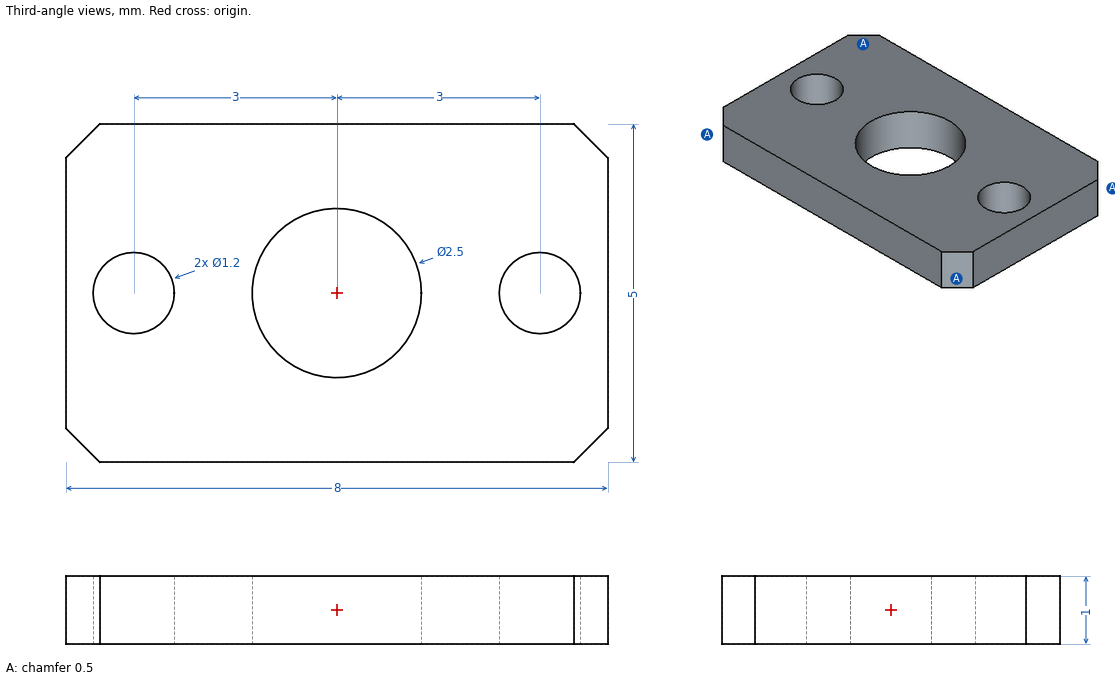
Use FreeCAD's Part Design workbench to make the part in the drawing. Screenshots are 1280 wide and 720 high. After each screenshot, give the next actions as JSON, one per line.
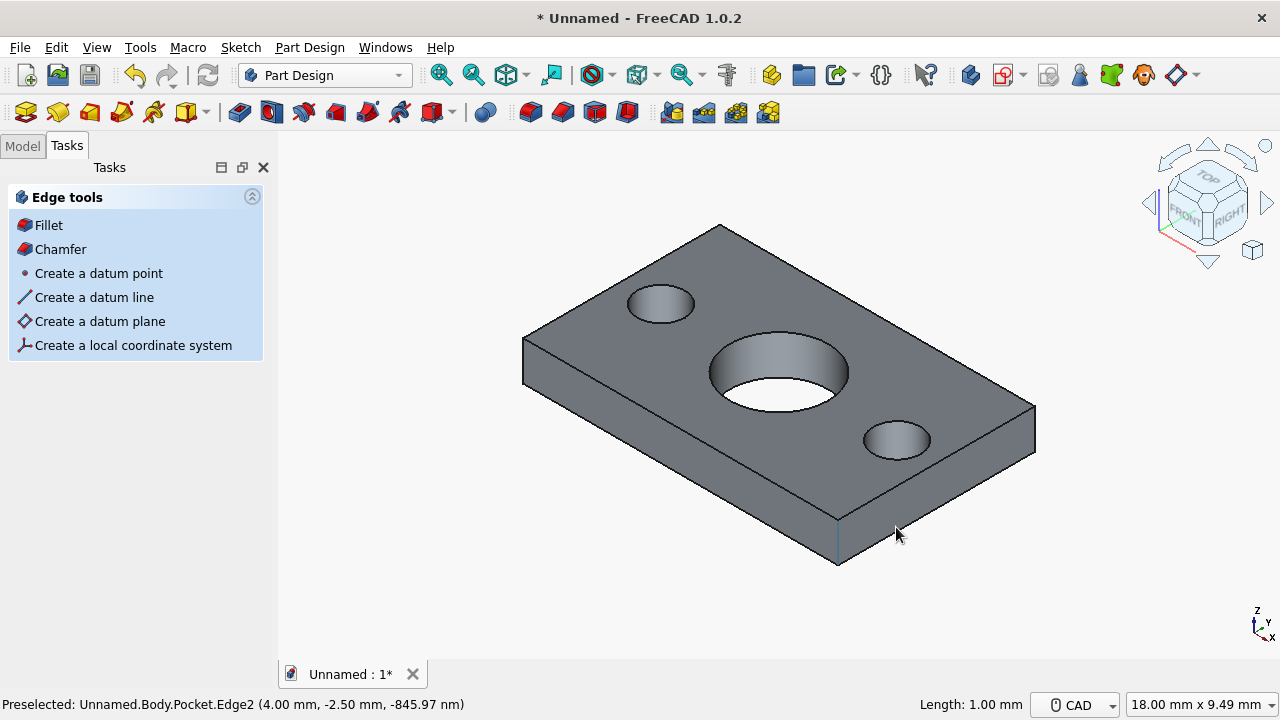
{"action": "key", "text": "2"}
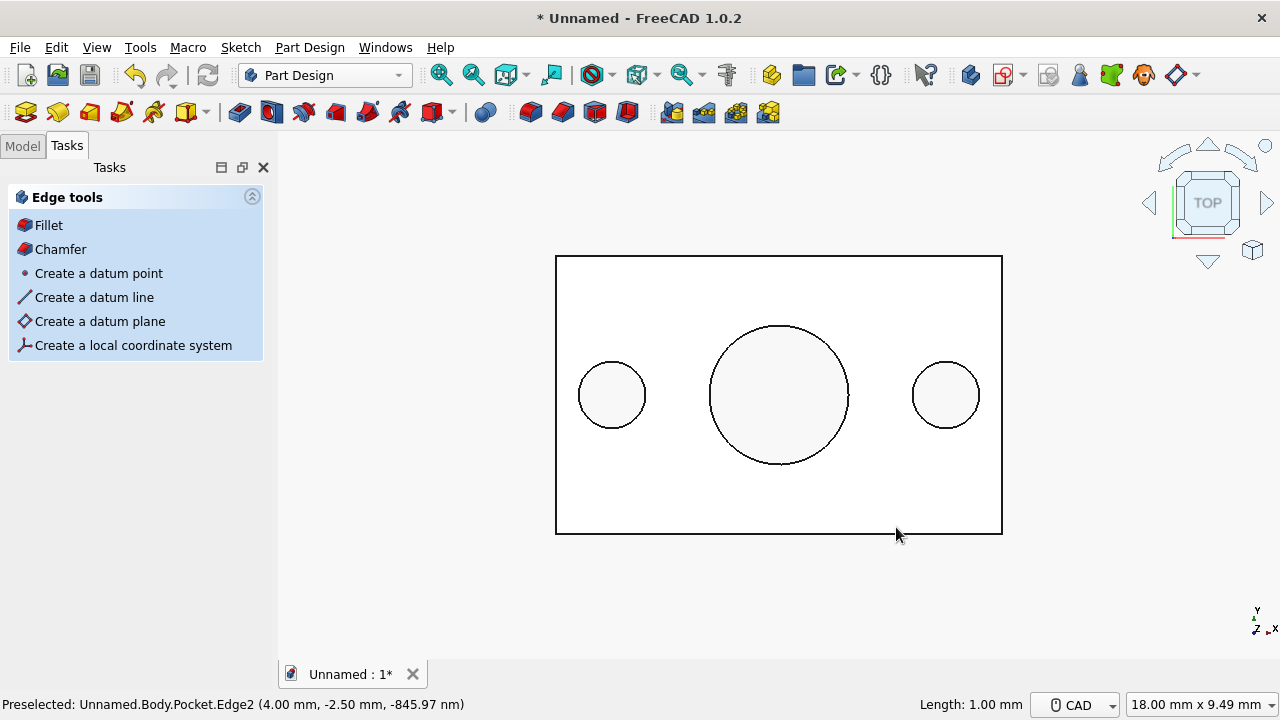
{"action": "key", "text": "1"}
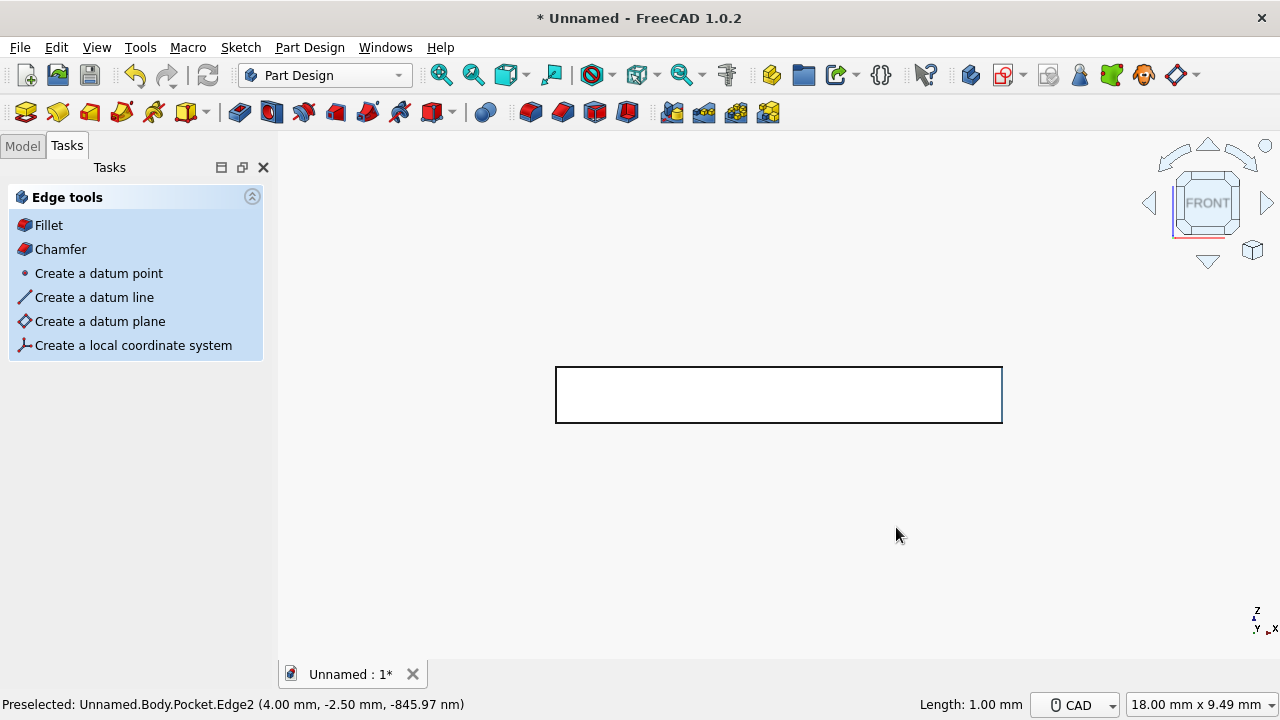
{"action": "left_click", "coordinate": [442, 76]}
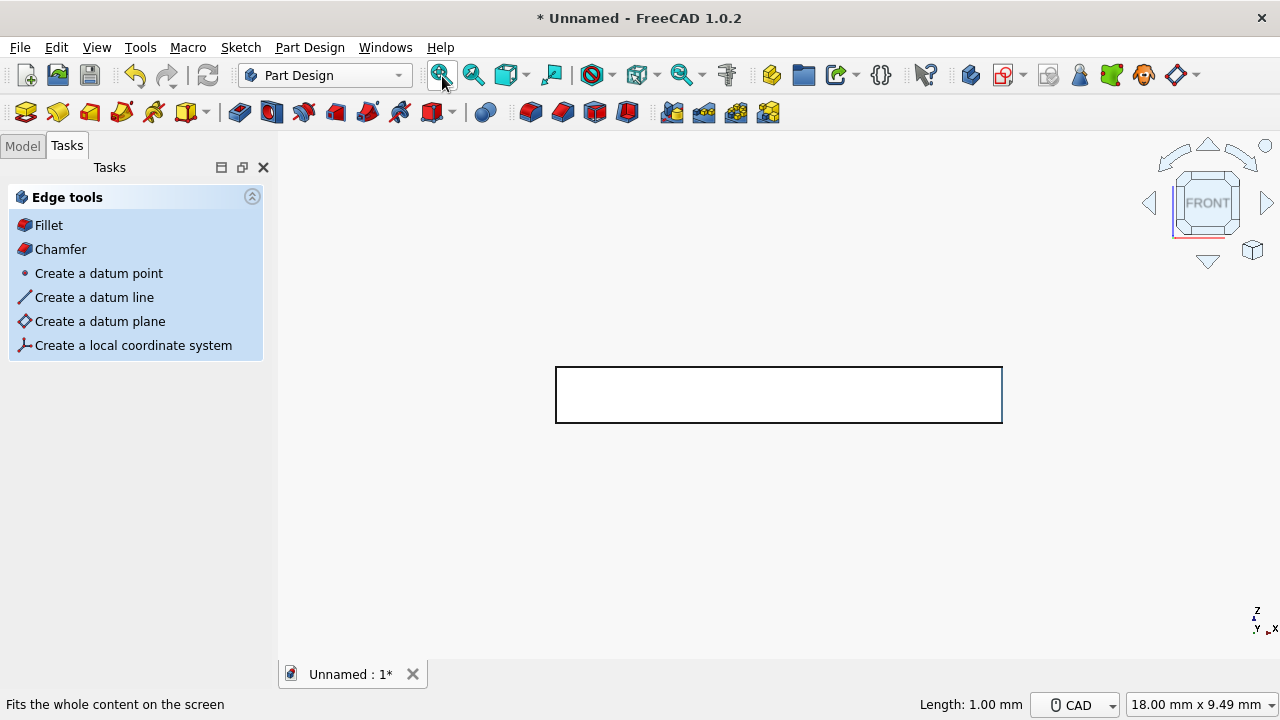
{"action": "left_click", "coordinate": [556, 394], "text": "ctrl"}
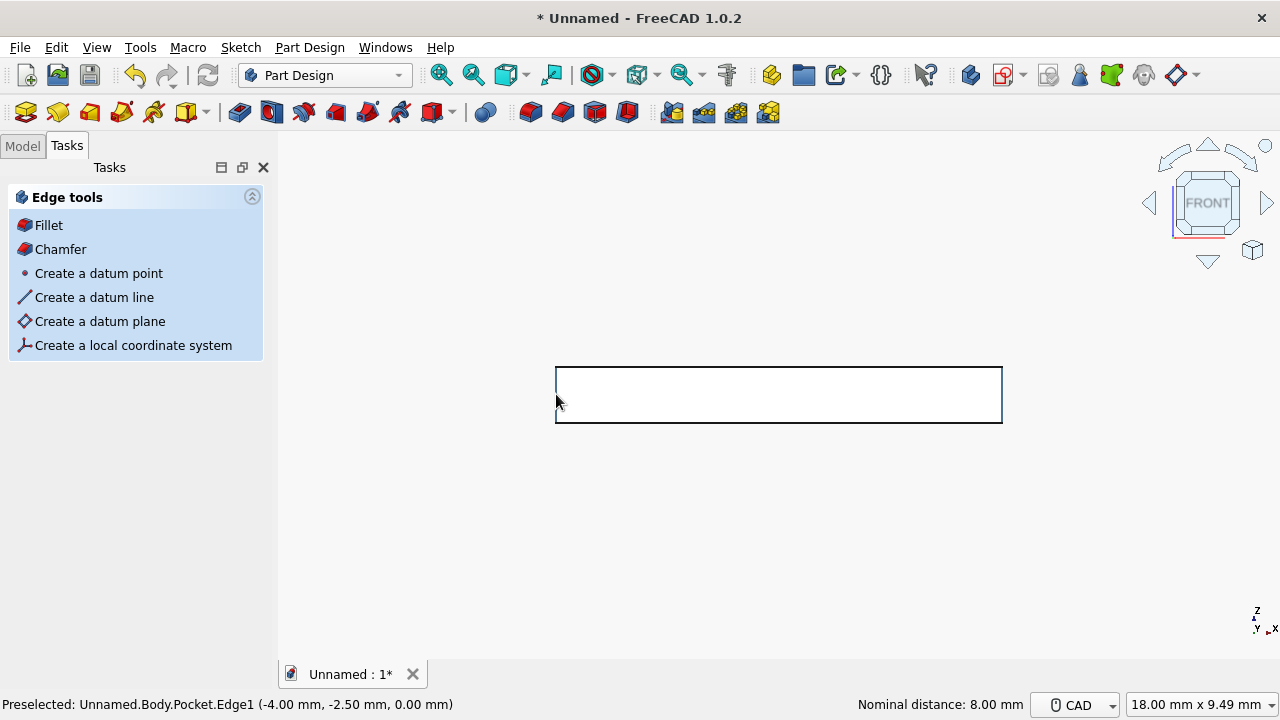
{"action": "key", "text": "3"}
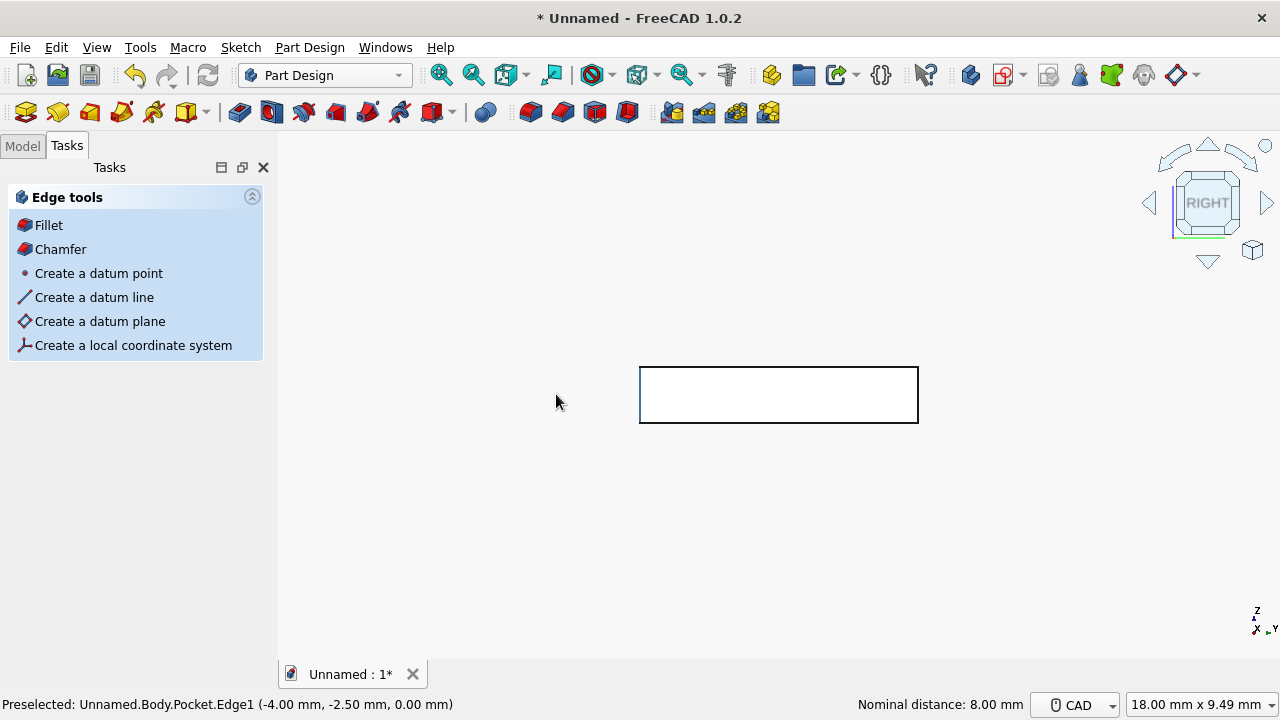
{"action": "left_click", "coordinate": [442, 76]}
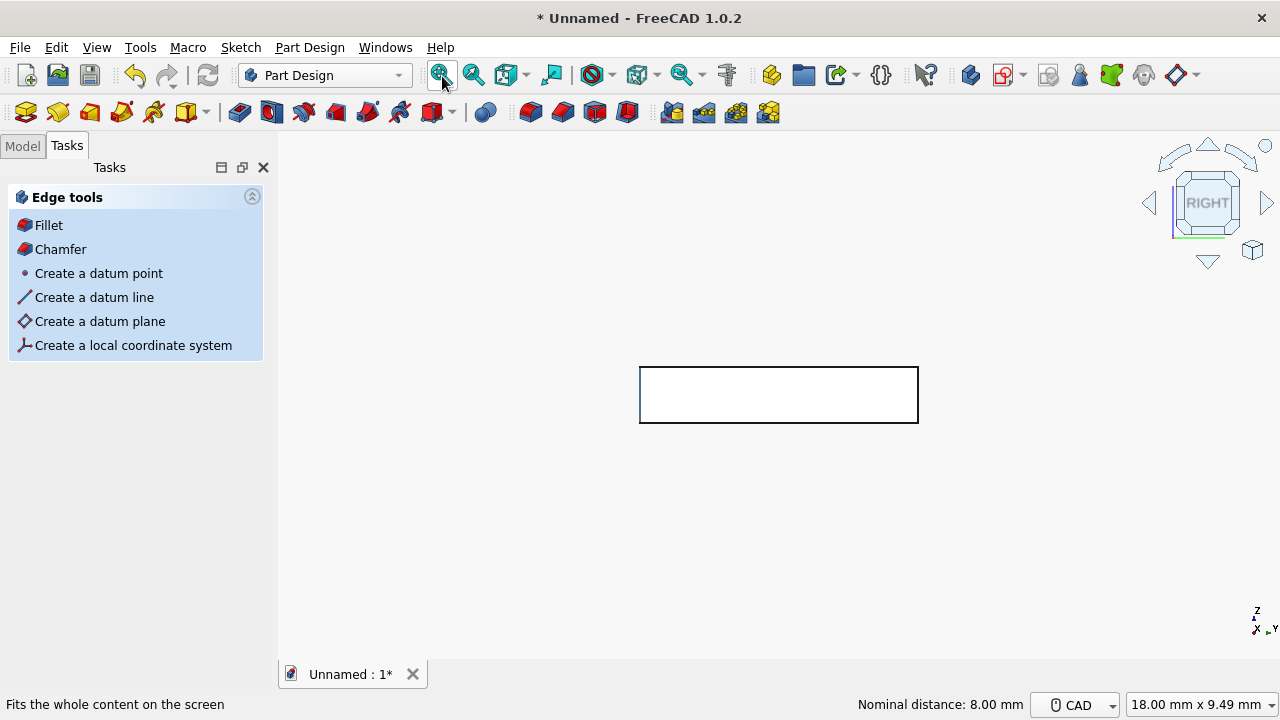
{"action": "left_click", "coordinate": [918, 394], "text": "ctrl"}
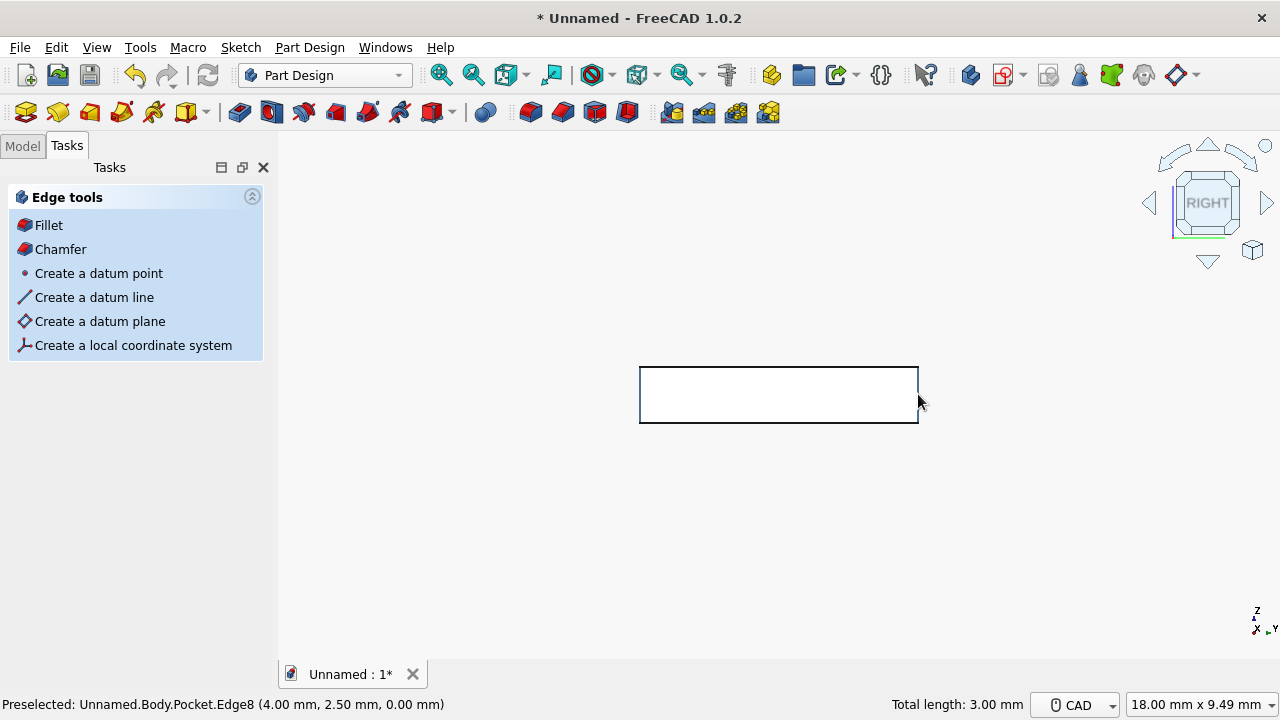
{"action": "key", "text": "5"}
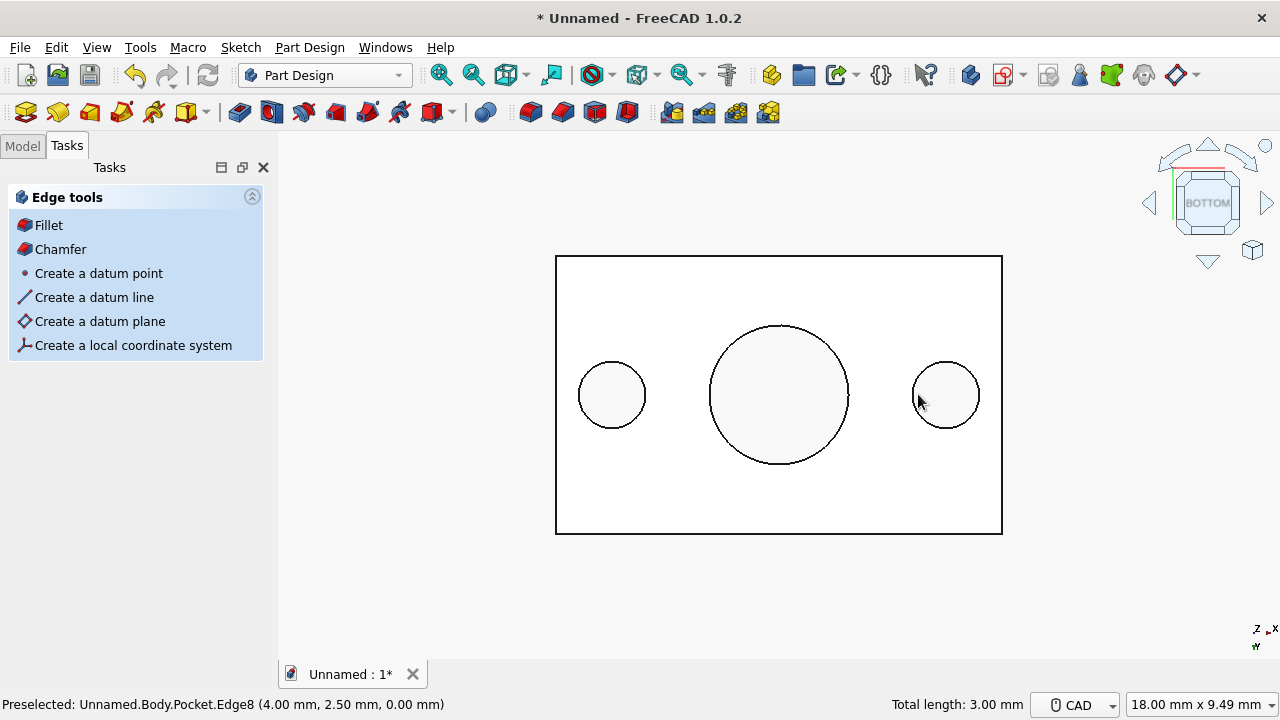
{"action": "key", "text": "4"}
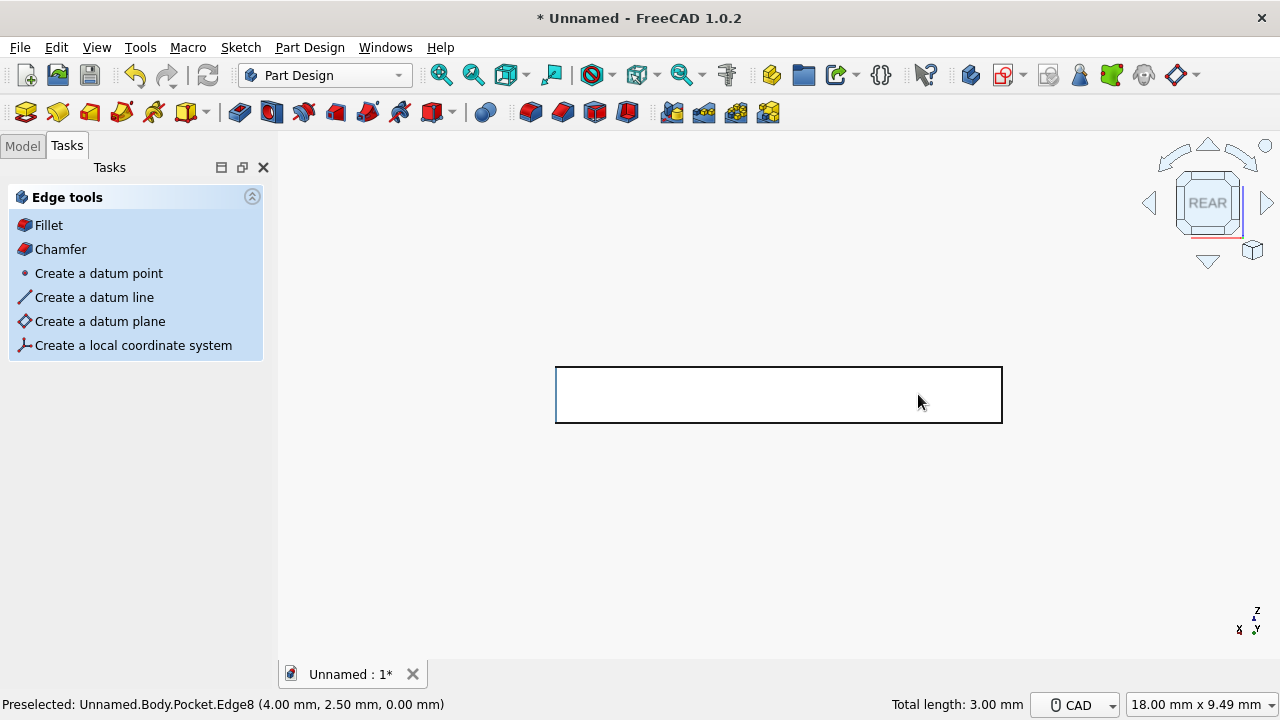
{"action": "left_click", "coordinate": [442, 76]}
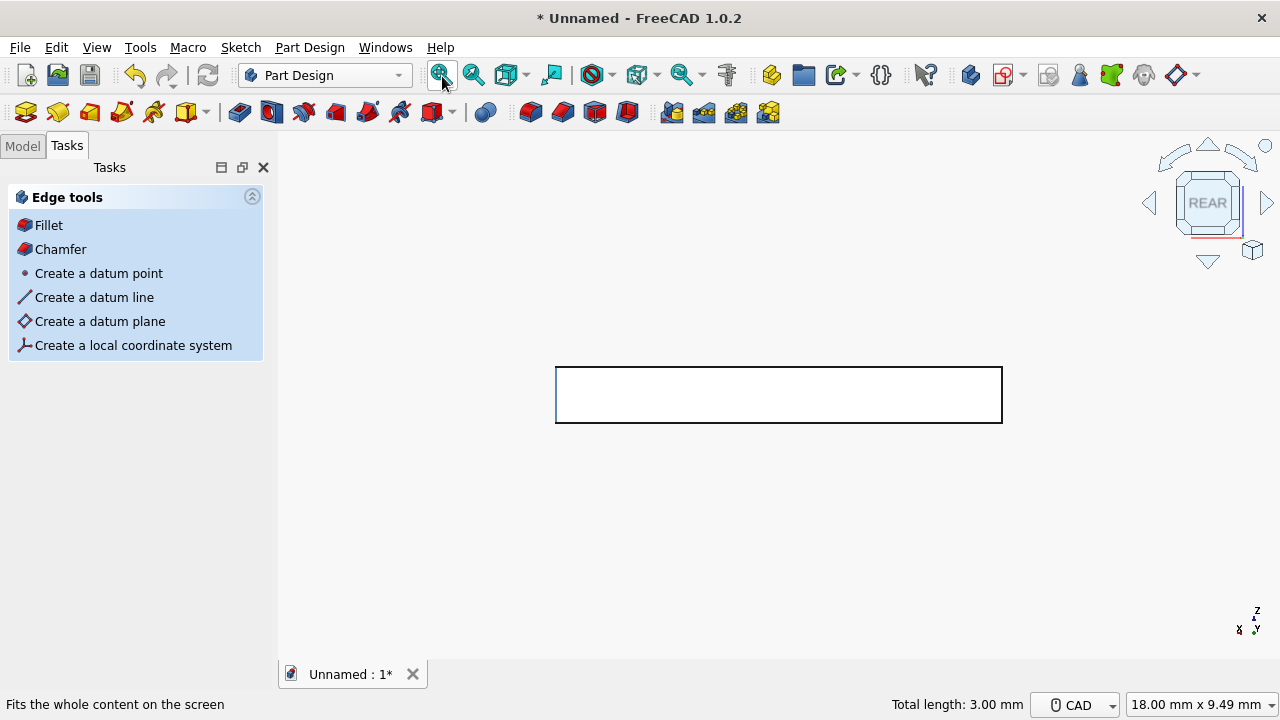
{"action": "left_click", "coordinate": [1002, 394], "text": "ctrl"}